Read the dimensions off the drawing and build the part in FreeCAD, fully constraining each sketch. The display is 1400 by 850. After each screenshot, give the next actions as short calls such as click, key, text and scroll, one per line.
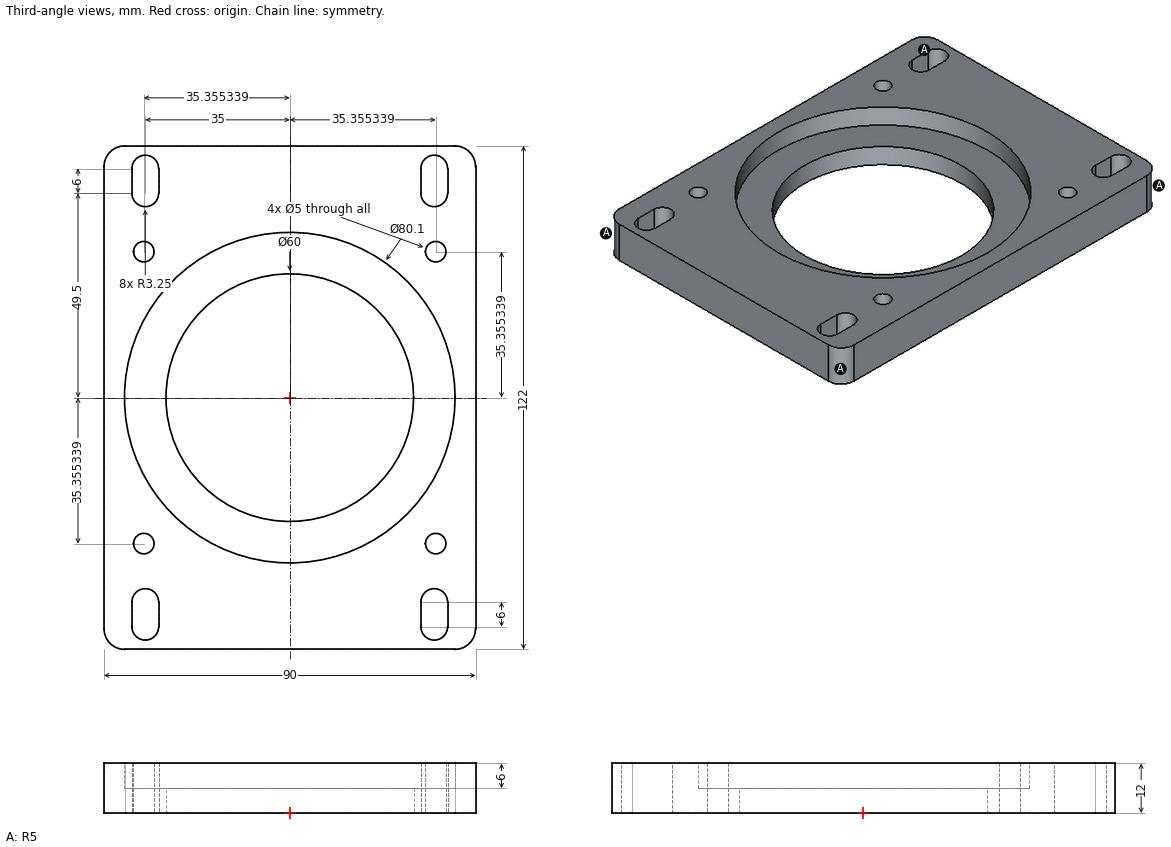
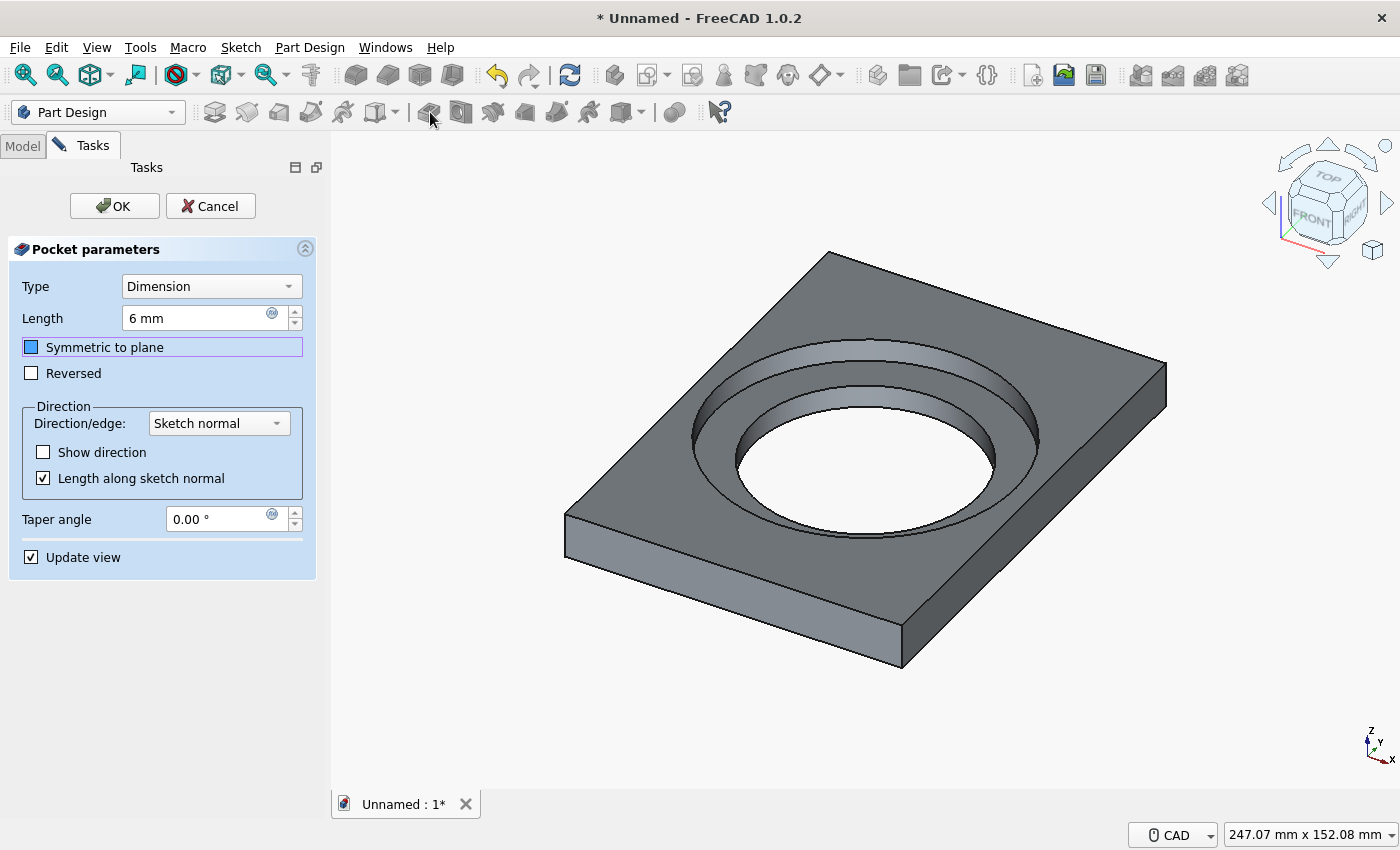
click(115, 206)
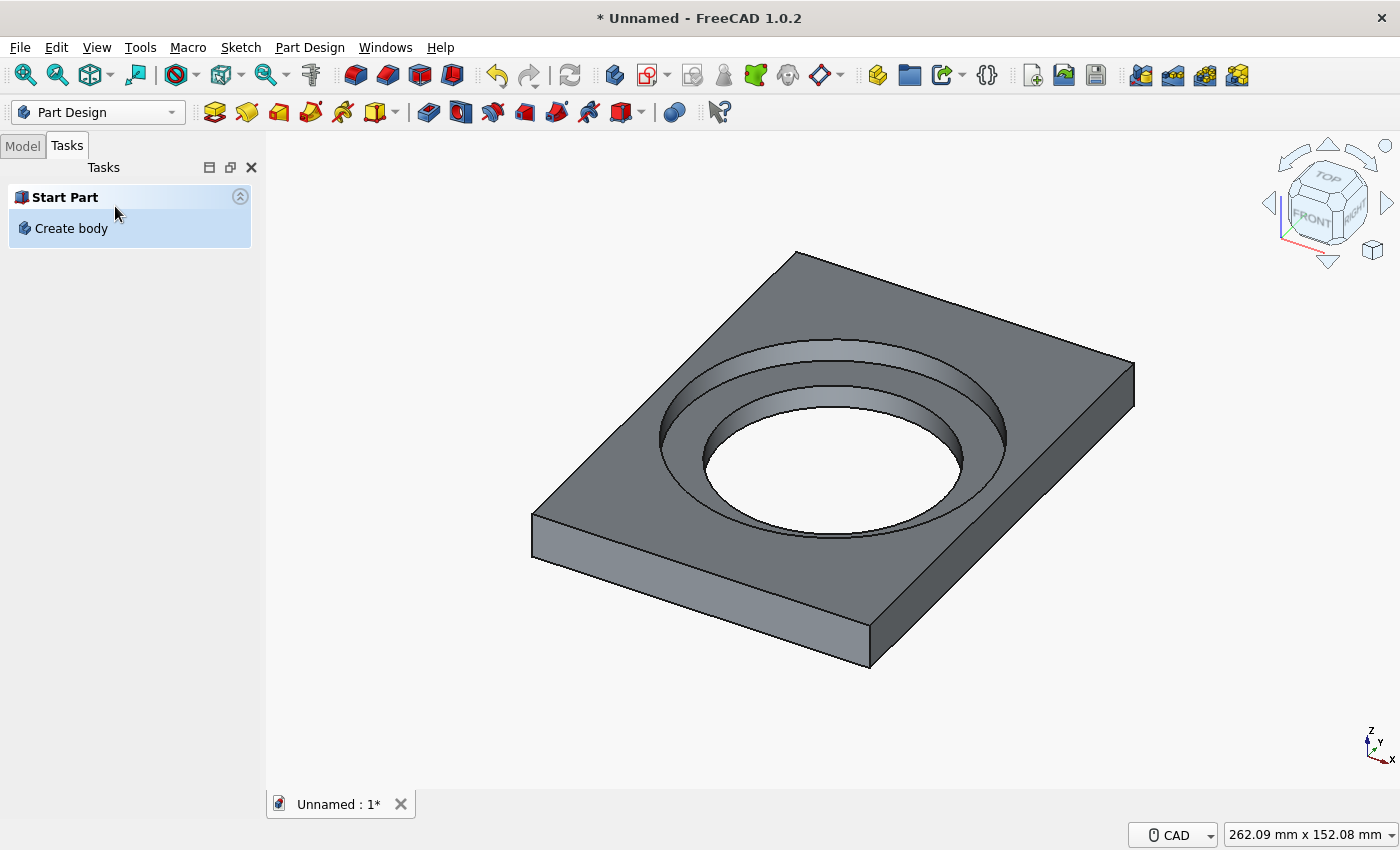
click(816, 582)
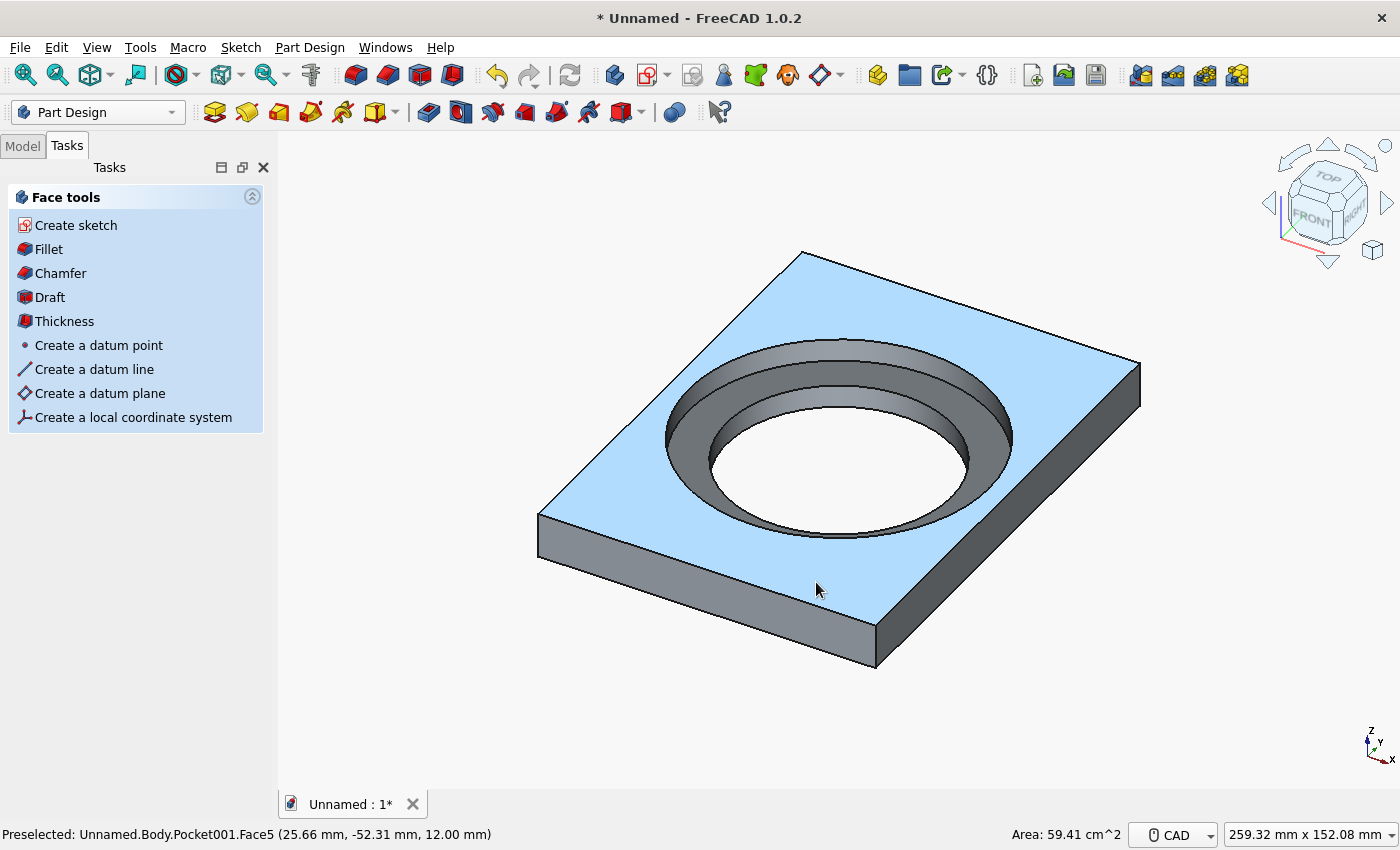
click(648, 76)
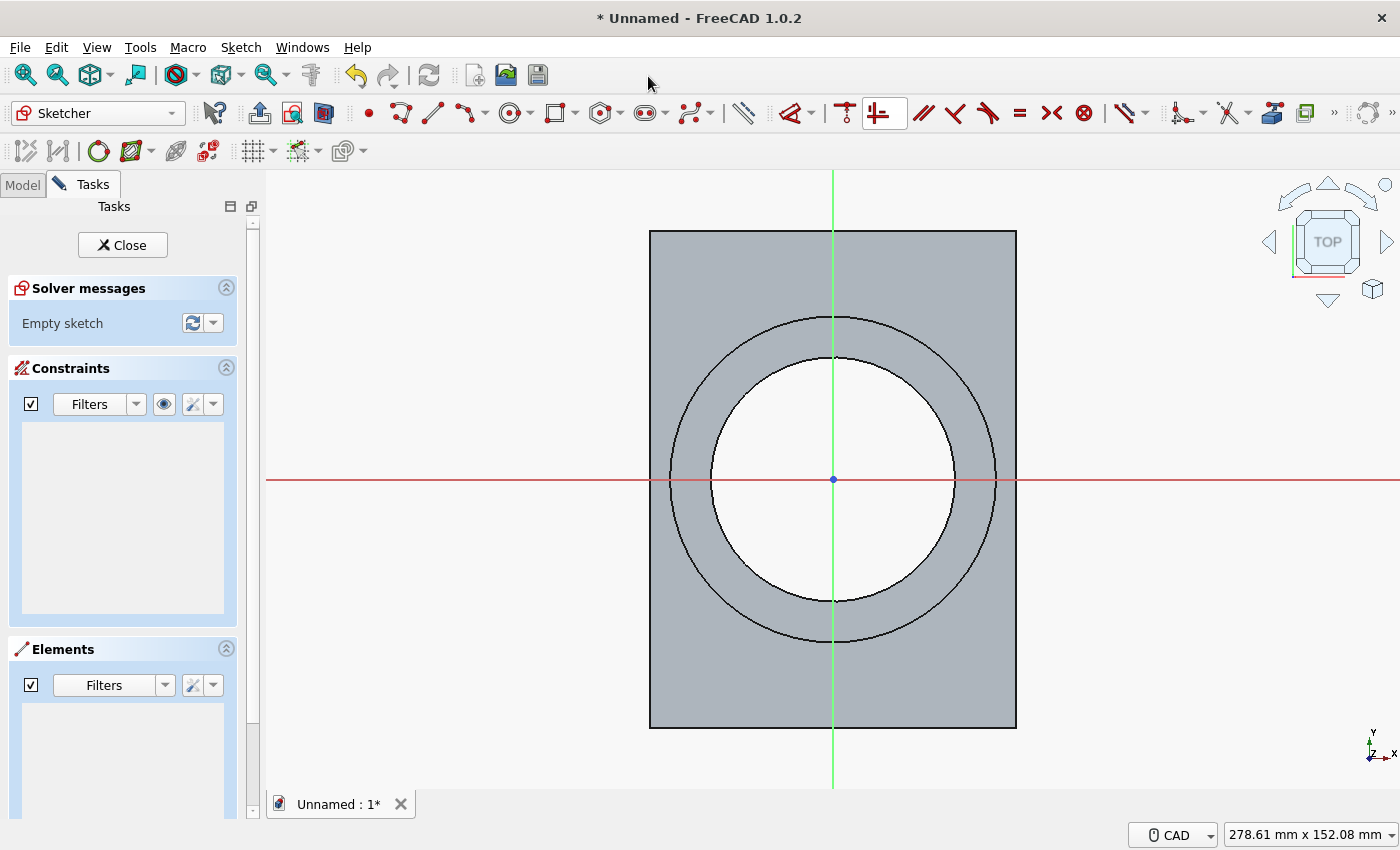
click(510, 114)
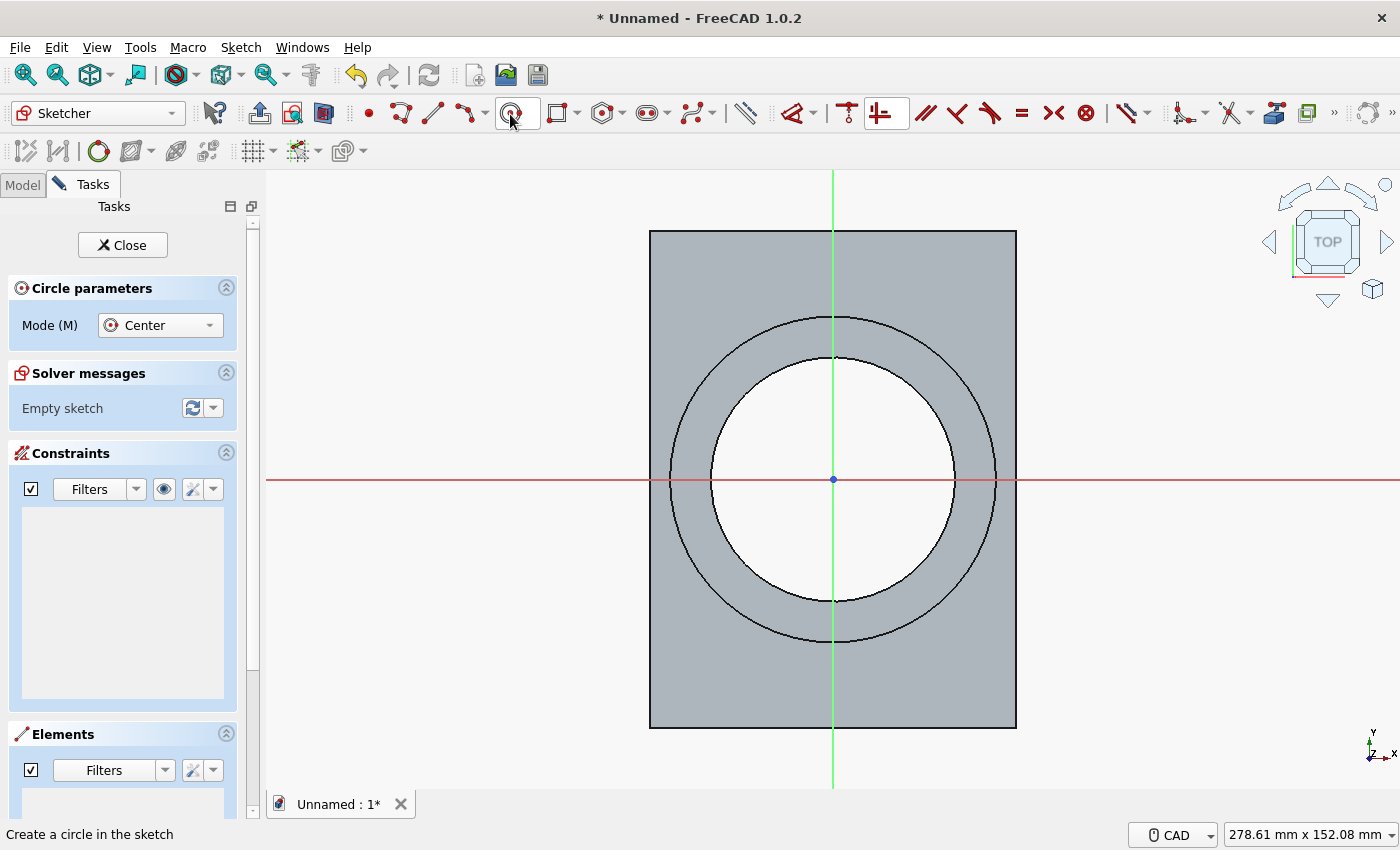
scroll(977, 336, up, 5)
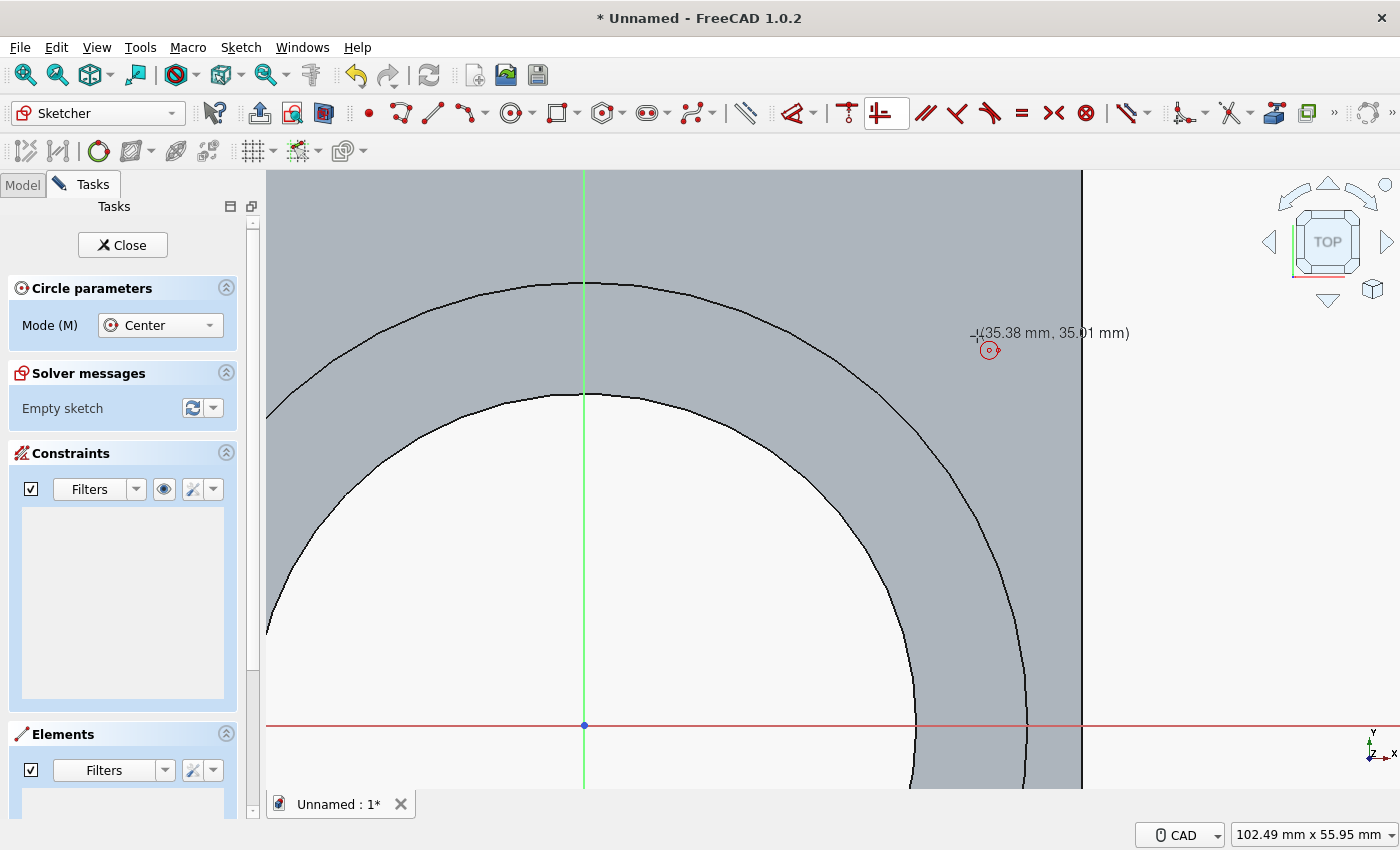
click(976, 334)
move(995, 315)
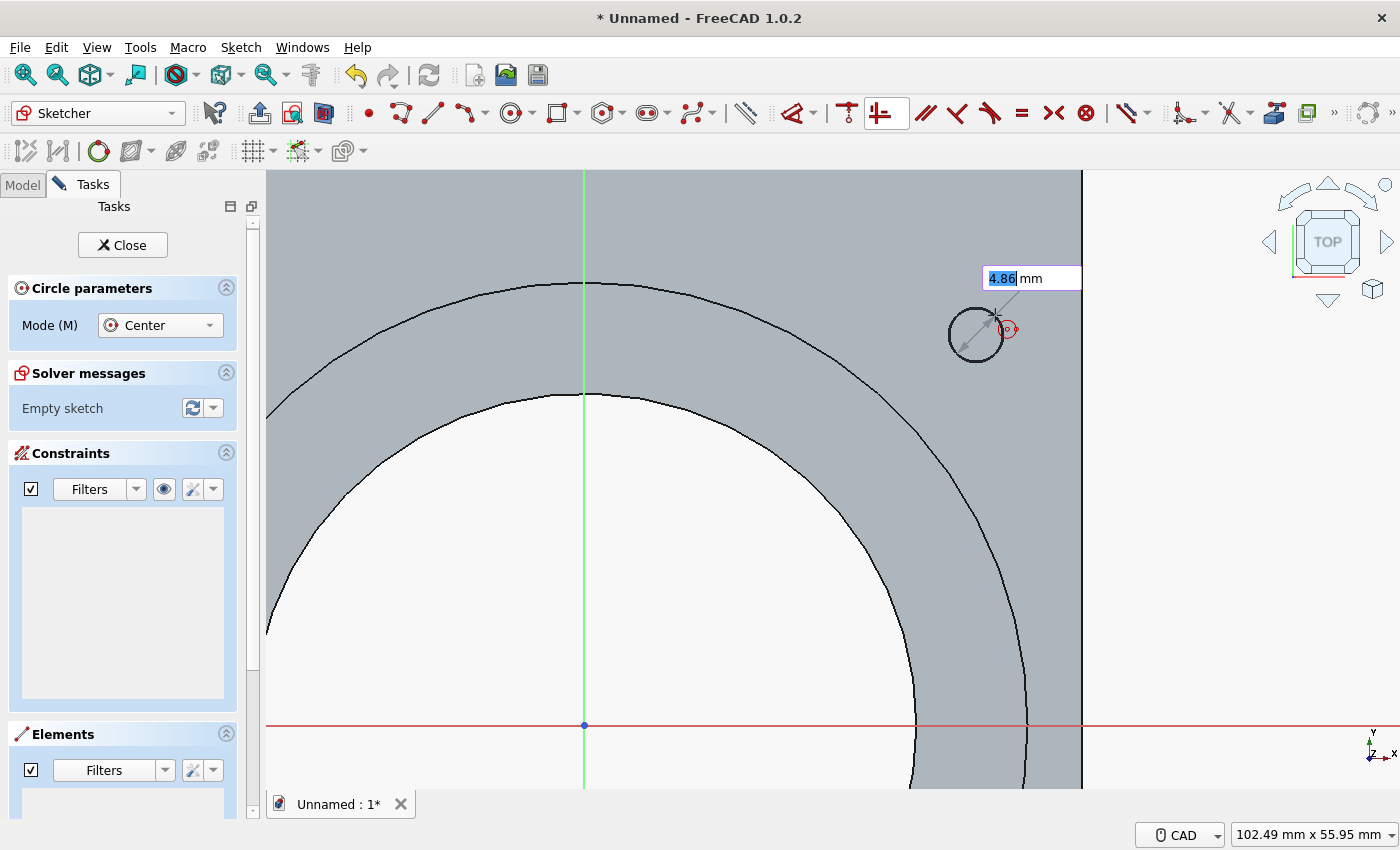
text(5)
key(Return)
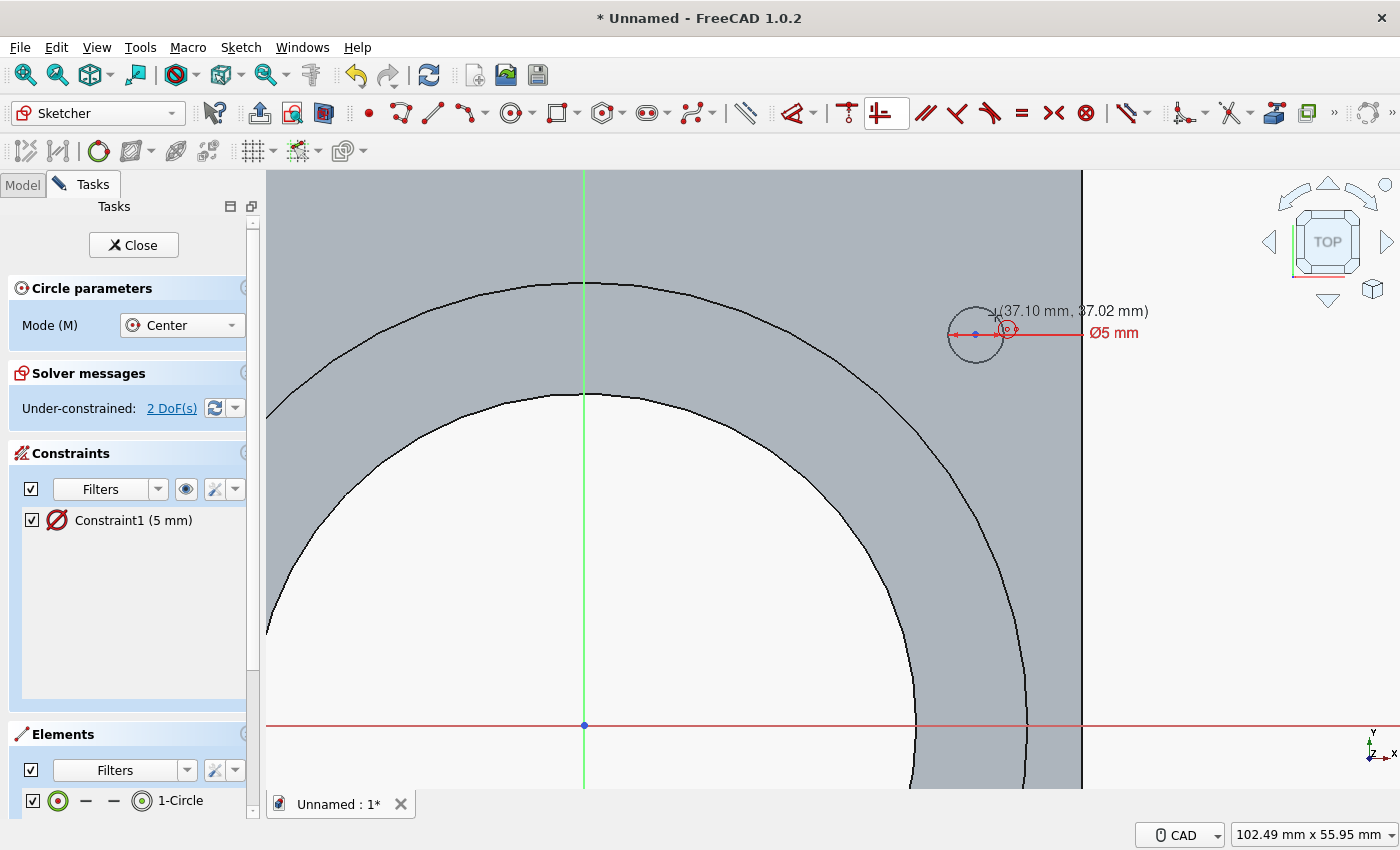
scroll(911, 279, down, 4)